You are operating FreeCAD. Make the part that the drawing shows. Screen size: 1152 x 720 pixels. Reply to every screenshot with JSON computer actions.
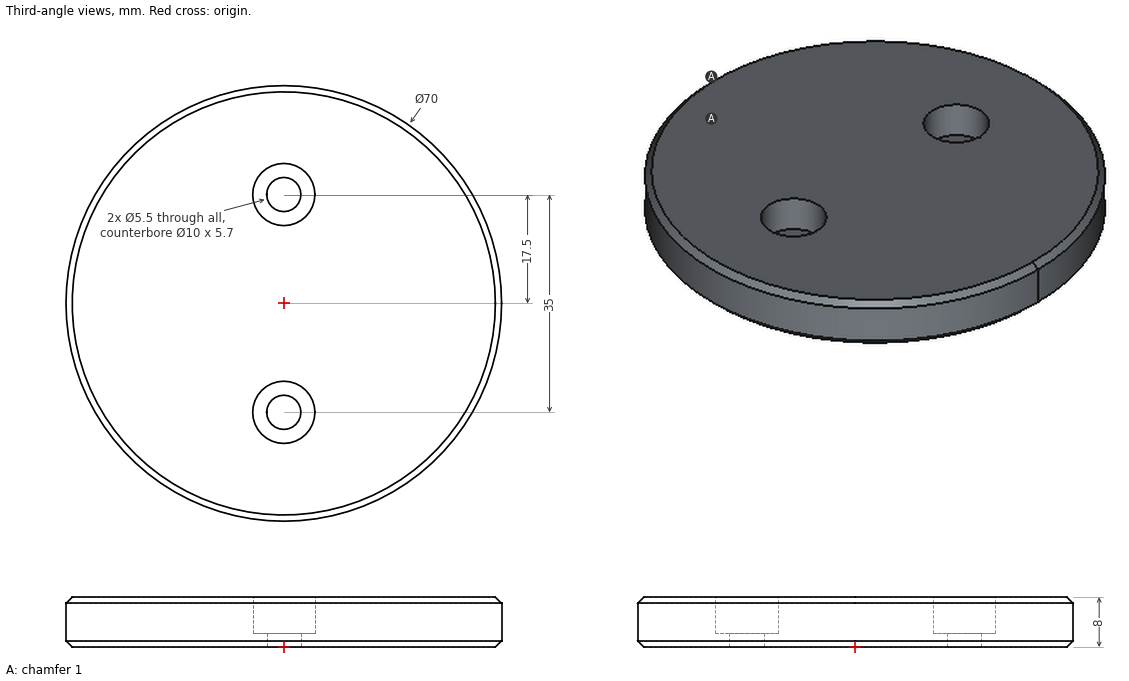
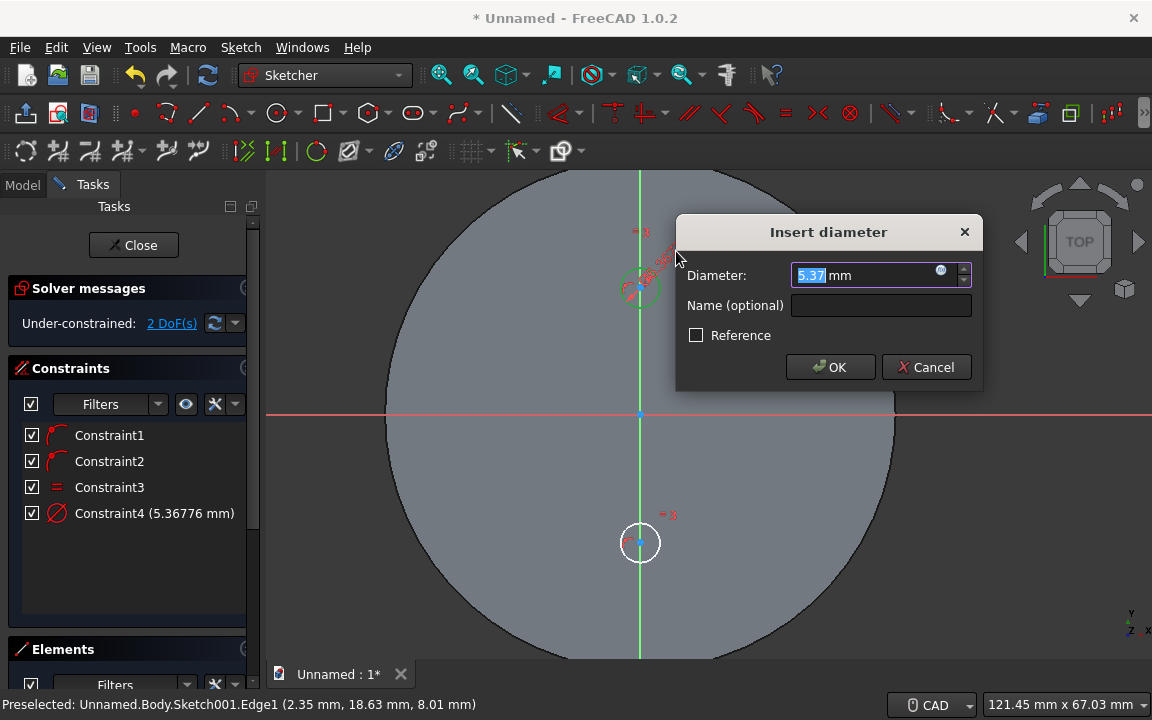
{"action": "type", "text": "5.5"}
{"action": "key", "text": "Return"}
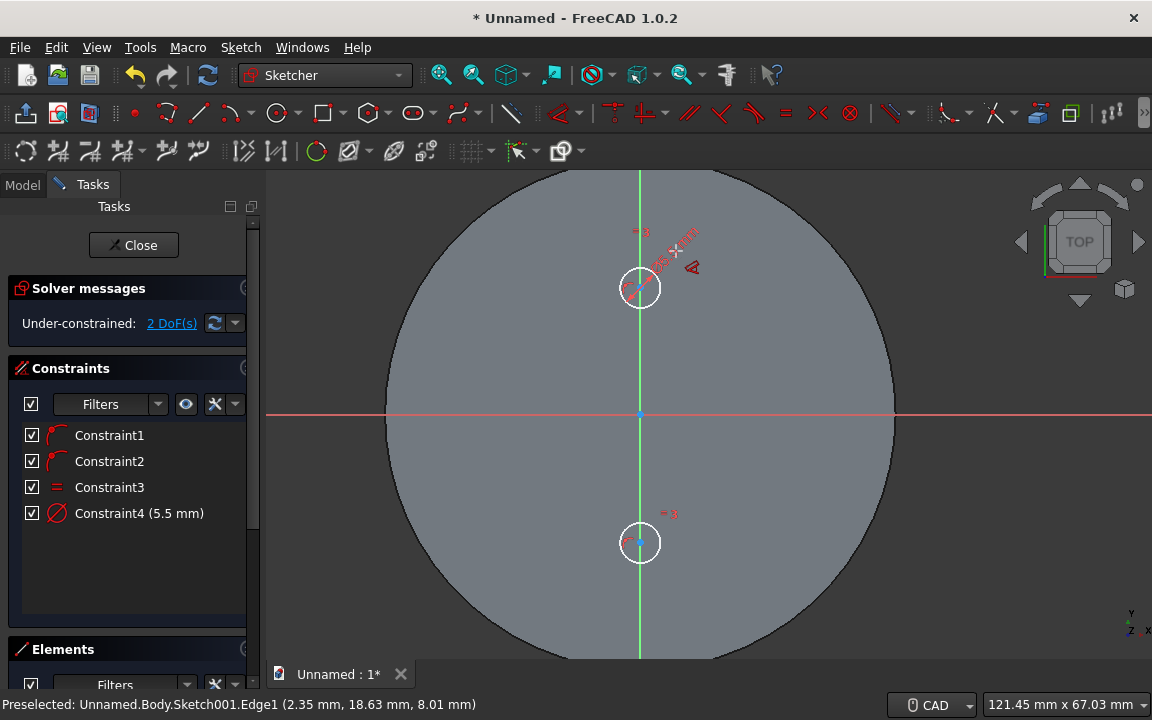
{"action": "left_click", "coordinate": [640, 288]}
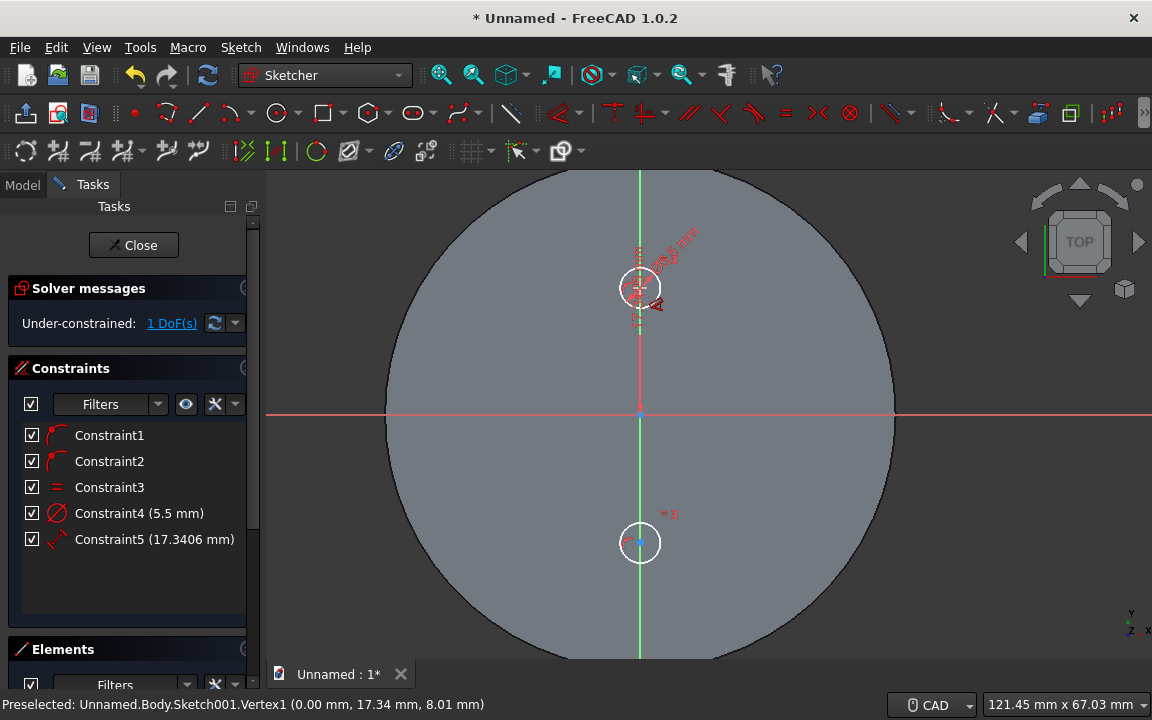
{"action": "left_click", "coordinate": [640, 543]}
{"action": "left_click", "coordinate": [674, 357]}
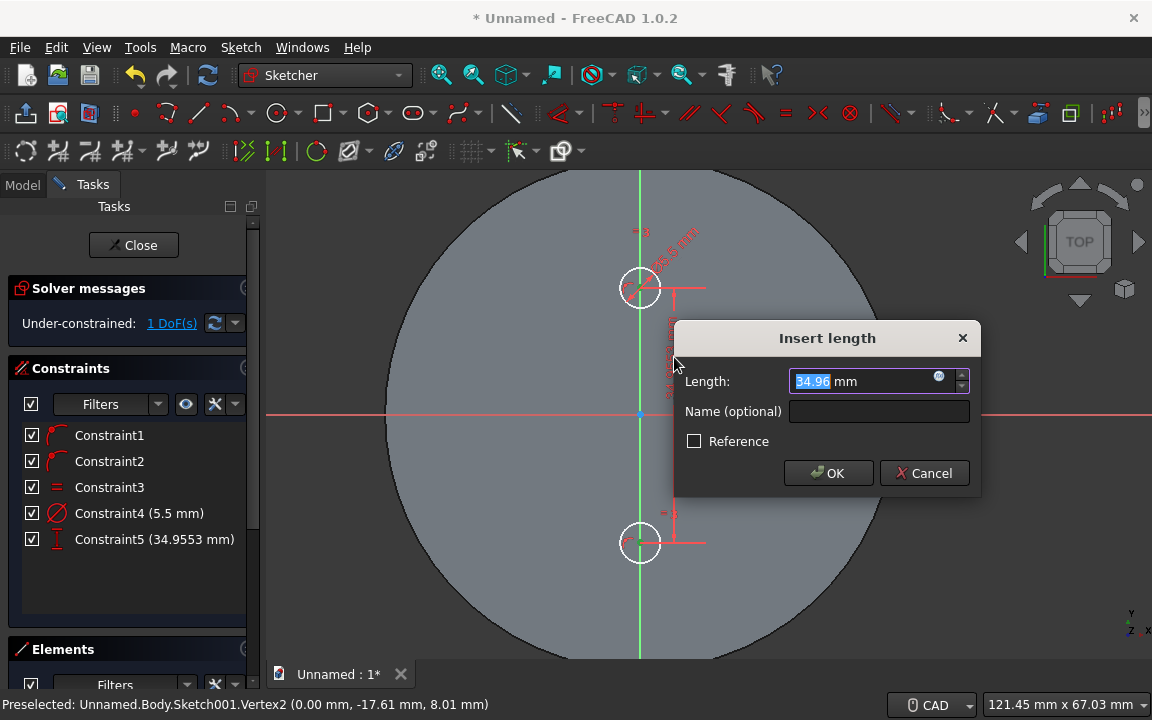
{"action": "type", "text": "35"}
{"action": "key", "text": "Return"}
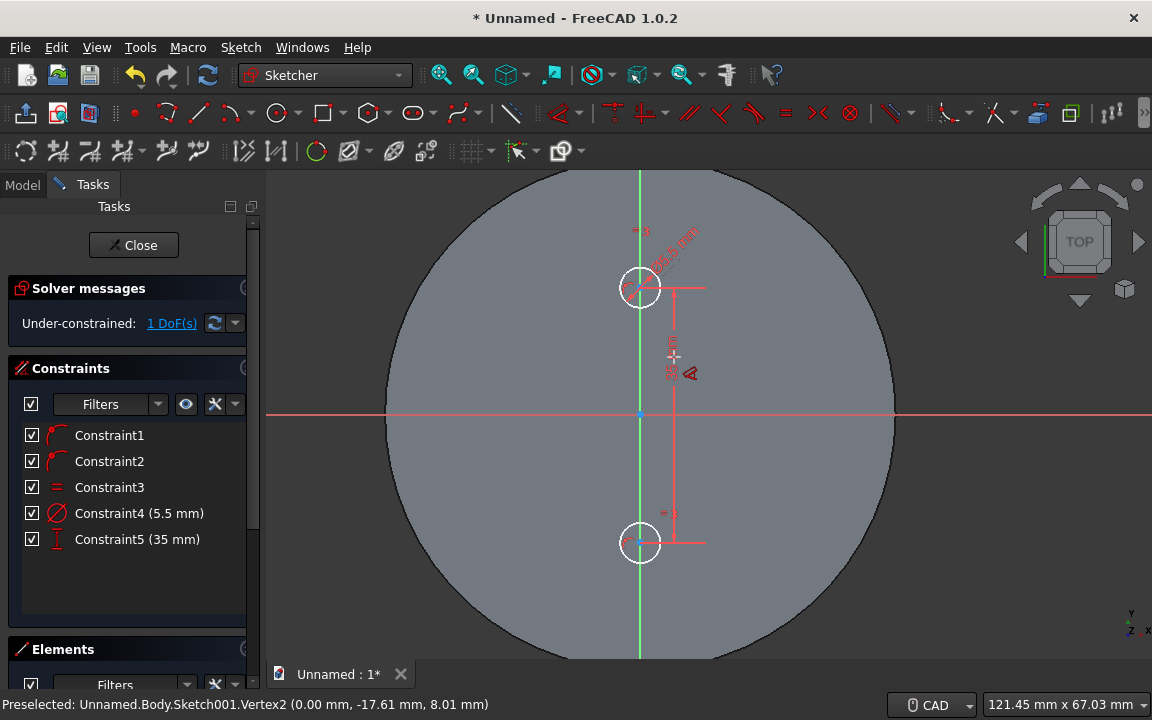
{"action": "left_click", "coordinate": [640, 288]}
{"action": "left_click", "coordinate": [674, 322]}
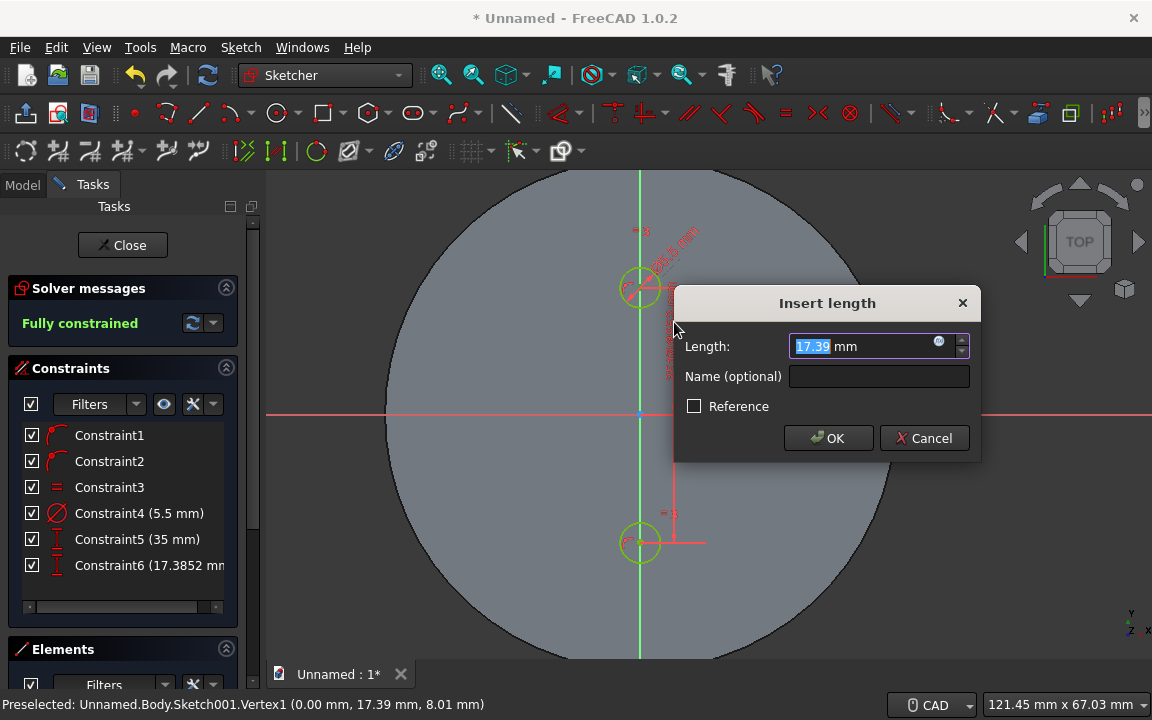
{"action": "type", "text": "17.5"}
{"action": "key", "text": "Return"}
{"action": "key", "text": "Escape"}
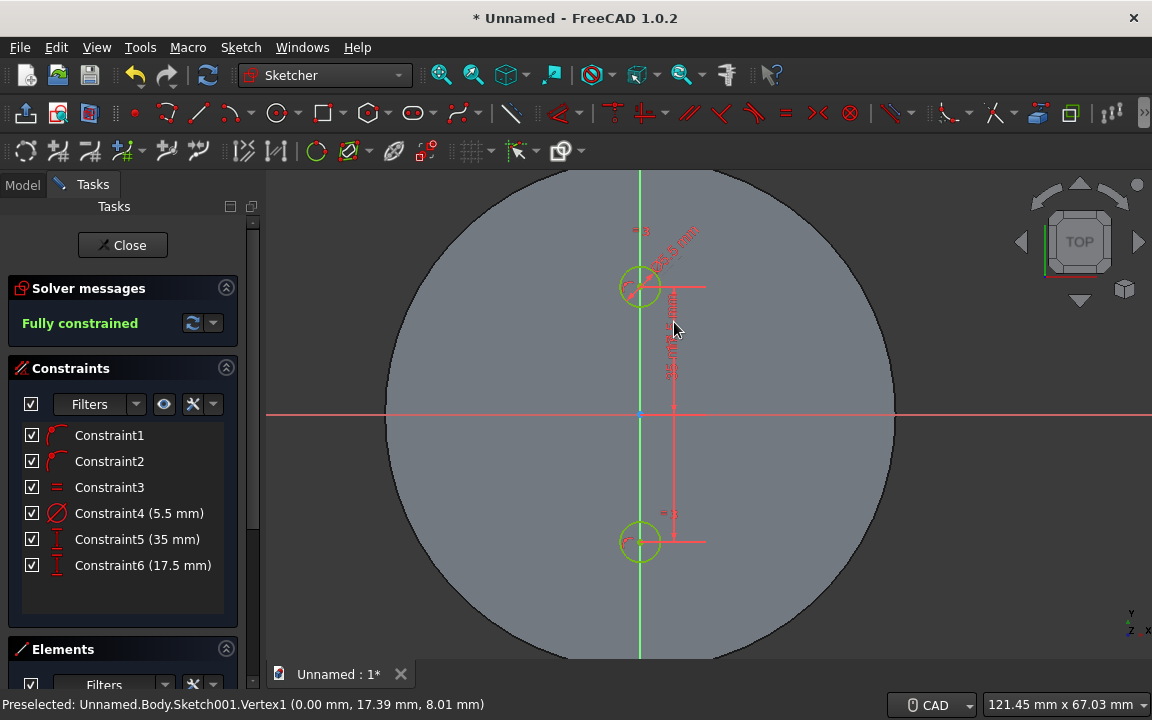
{"action": "left_click", "coordinate": [123, 245]}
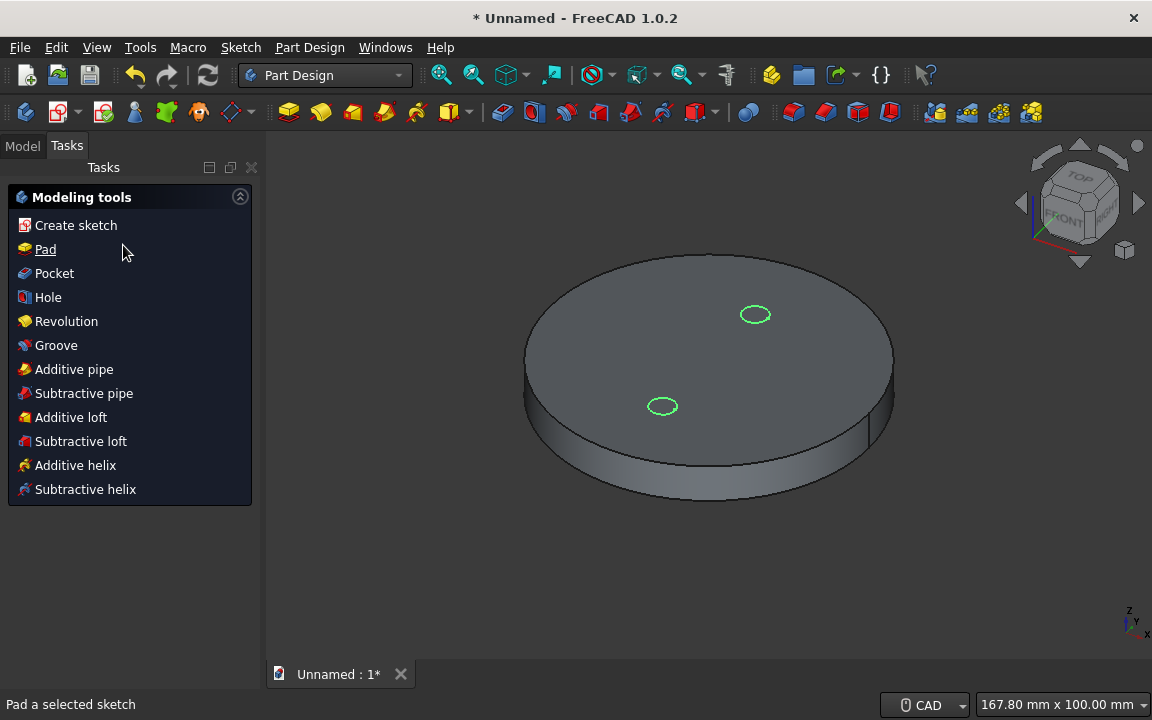
{"action": "left_click", "coordinate": [536, 112]}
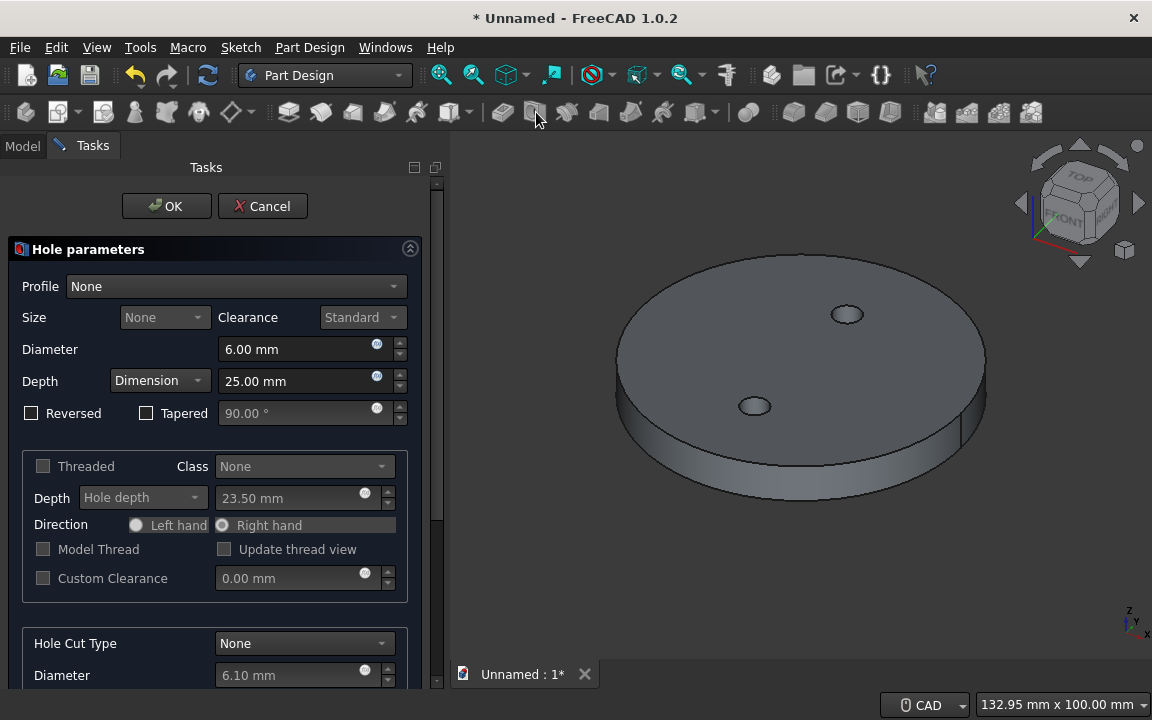
{"action": "triple_click", "coordinate": [305, 349]}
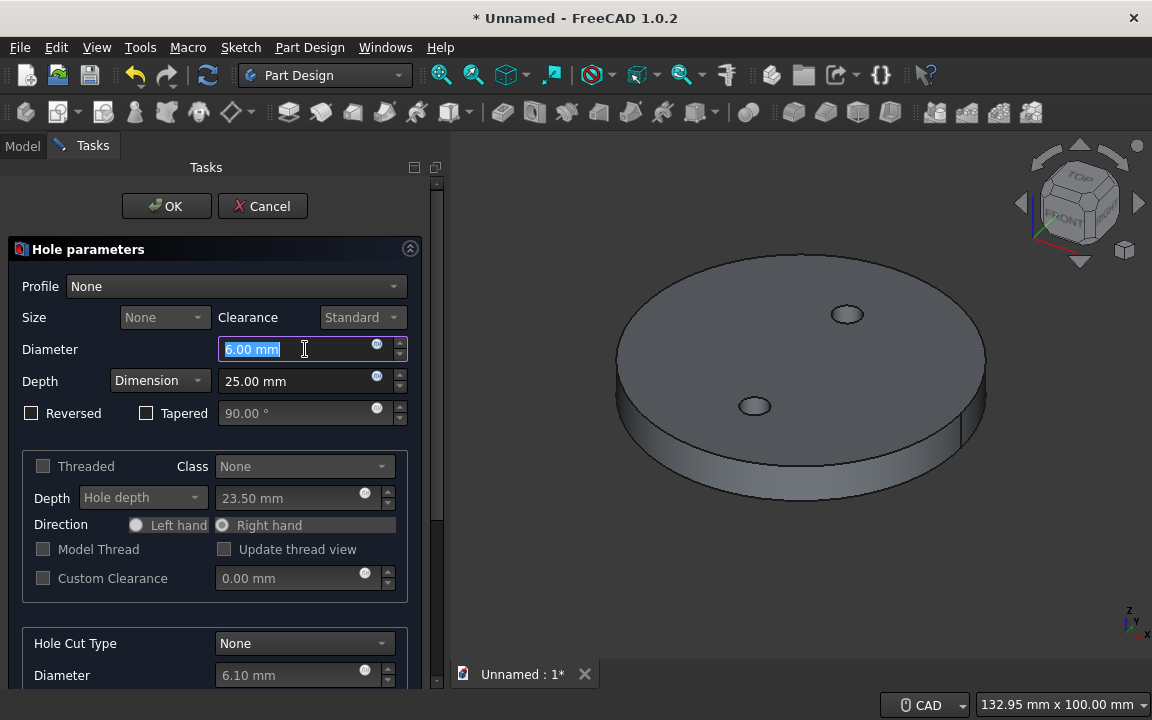
{"action": "type", "text": "5.5"}
{"action": "key", "text": "Tab"}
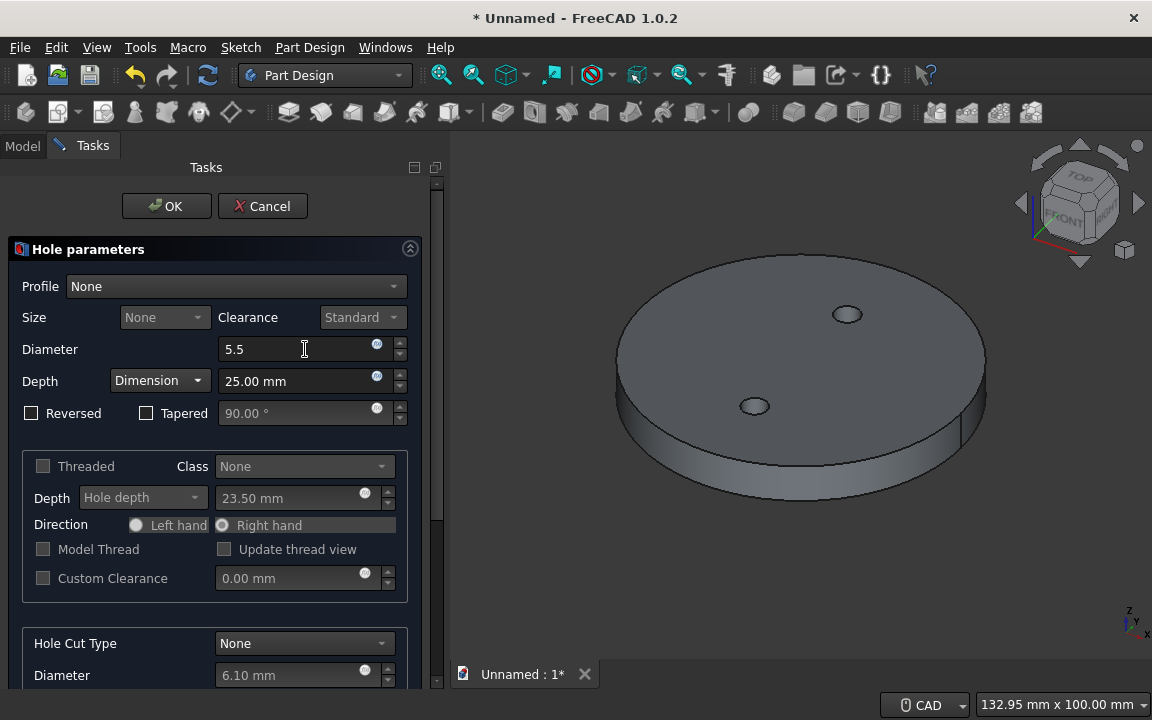
{"action": "left_click", "coordinate": [161, 380]}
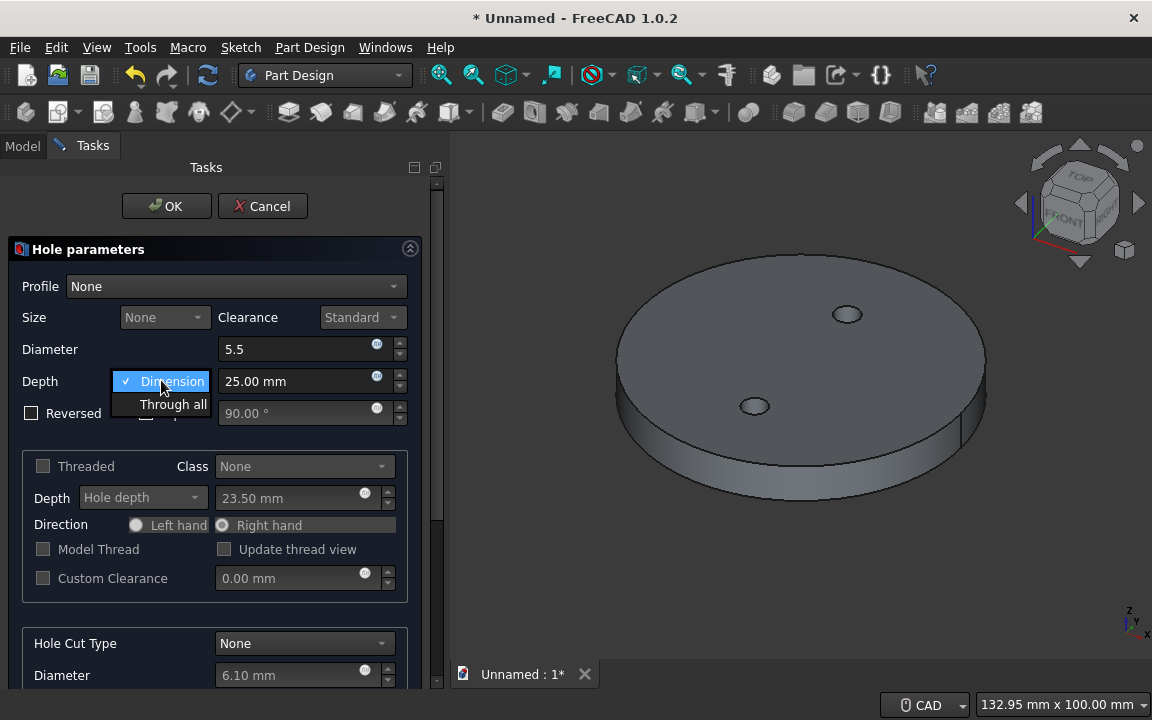
{"action": "left_click", "coordinate": [160, 404]}